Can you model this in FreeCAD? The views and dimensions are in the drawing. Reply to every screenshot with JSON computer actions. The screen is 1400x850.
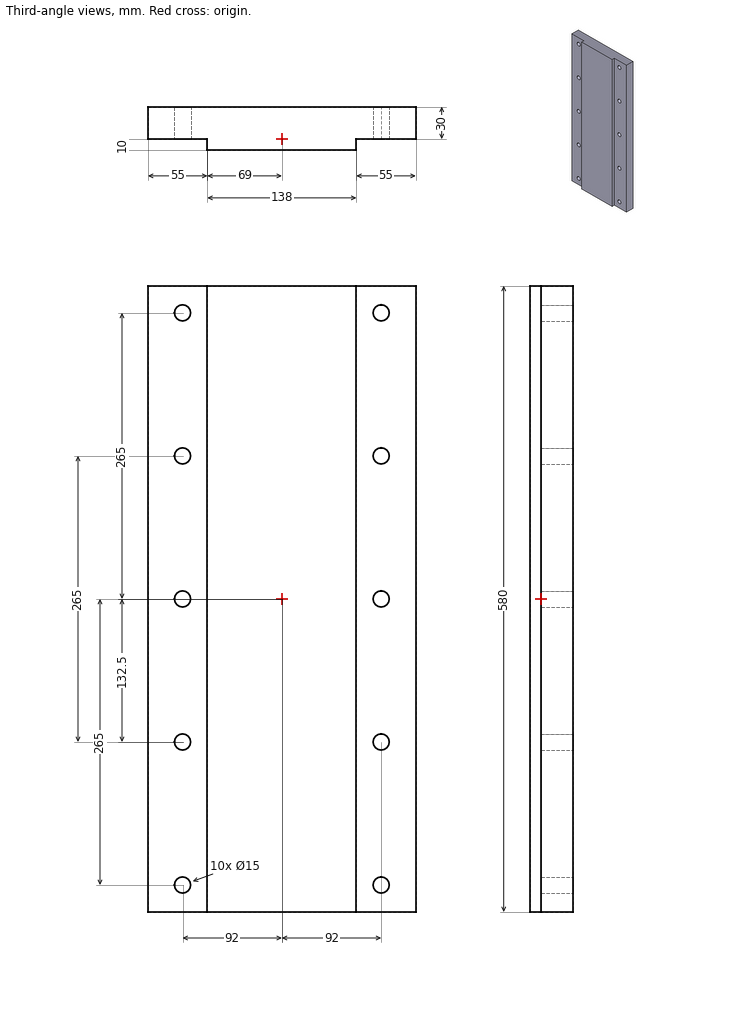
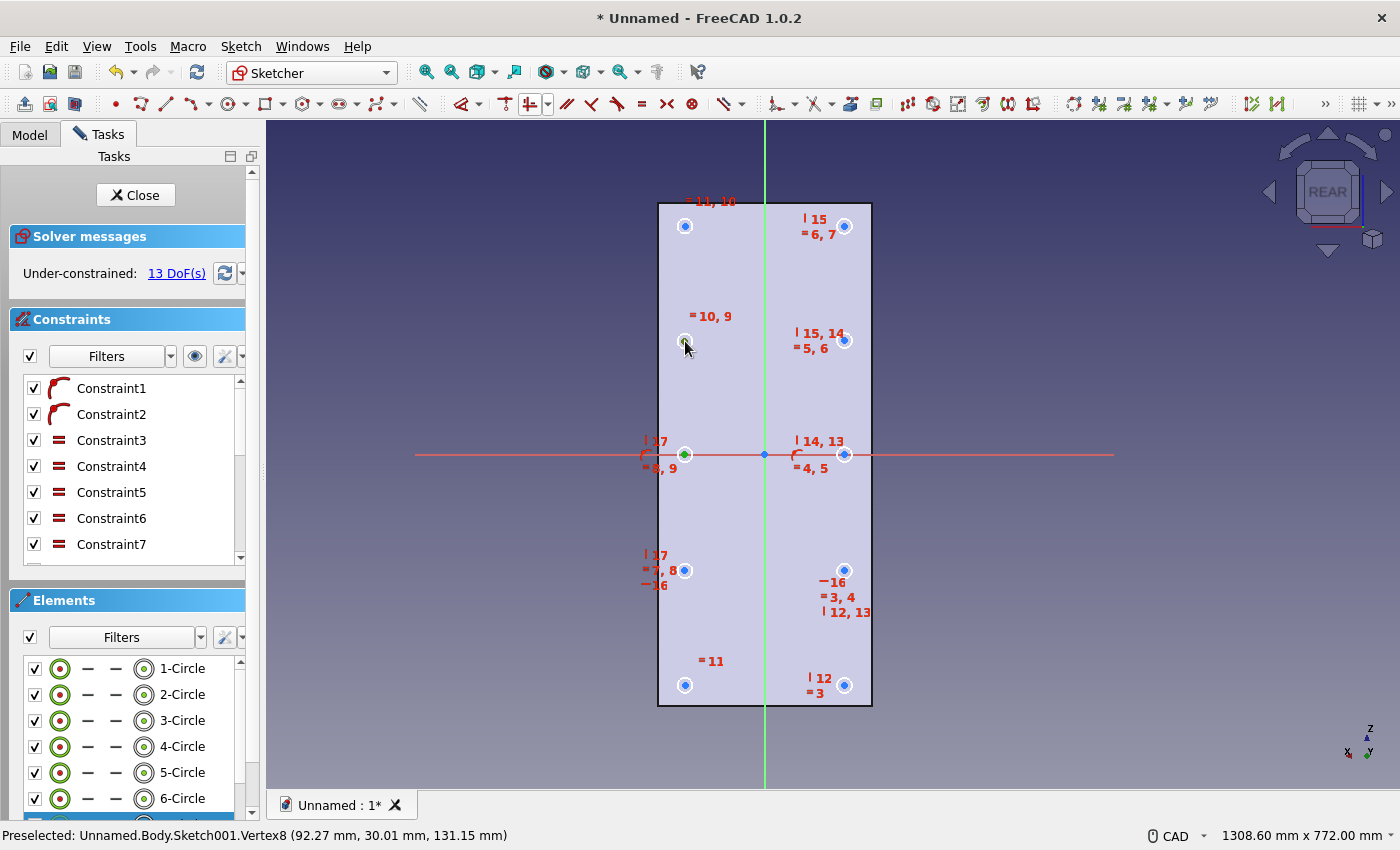
{"action": "left_click", "coordinate": [548, 104]}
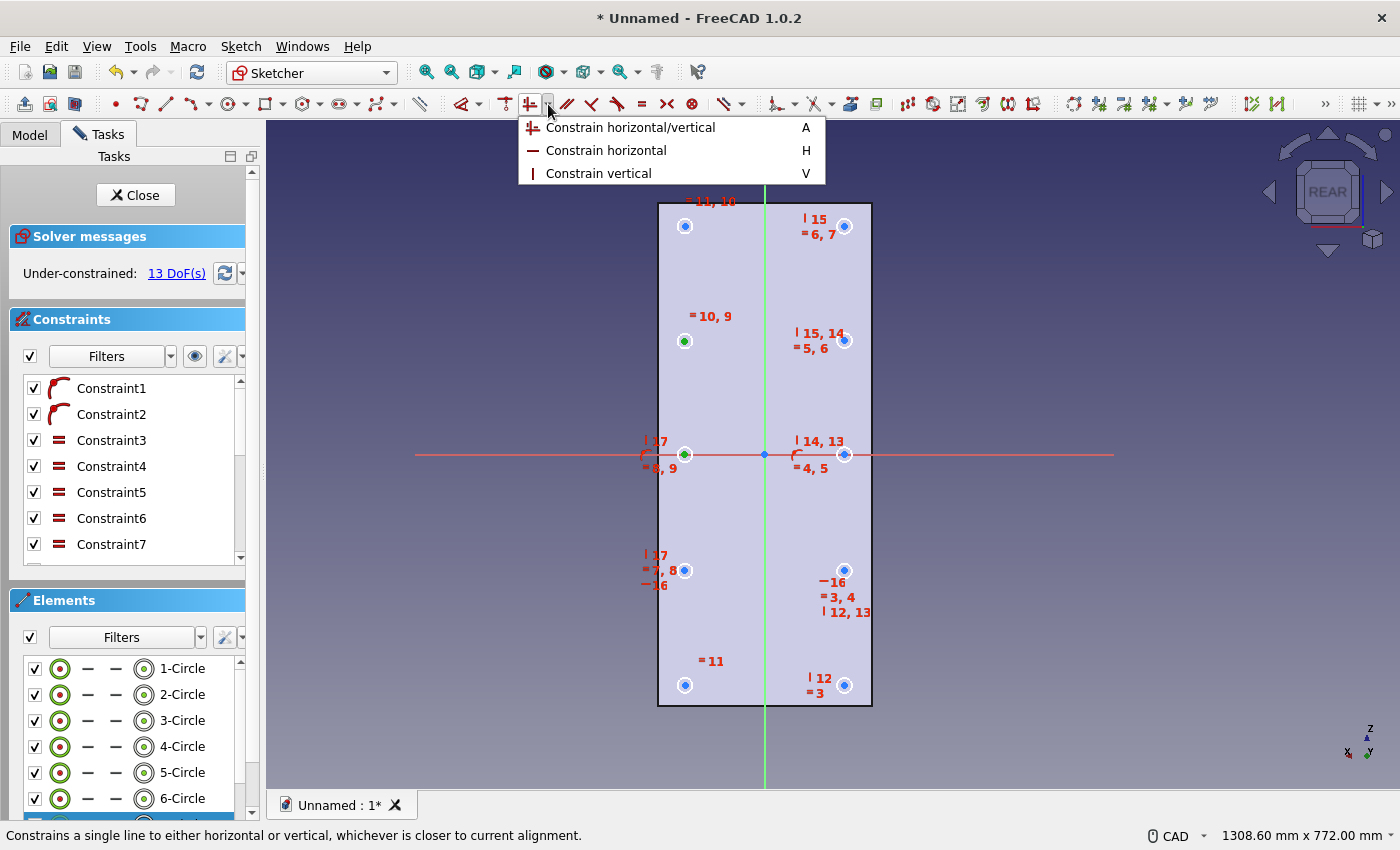
{"action": "left_click", "coordinate": [672, 174]}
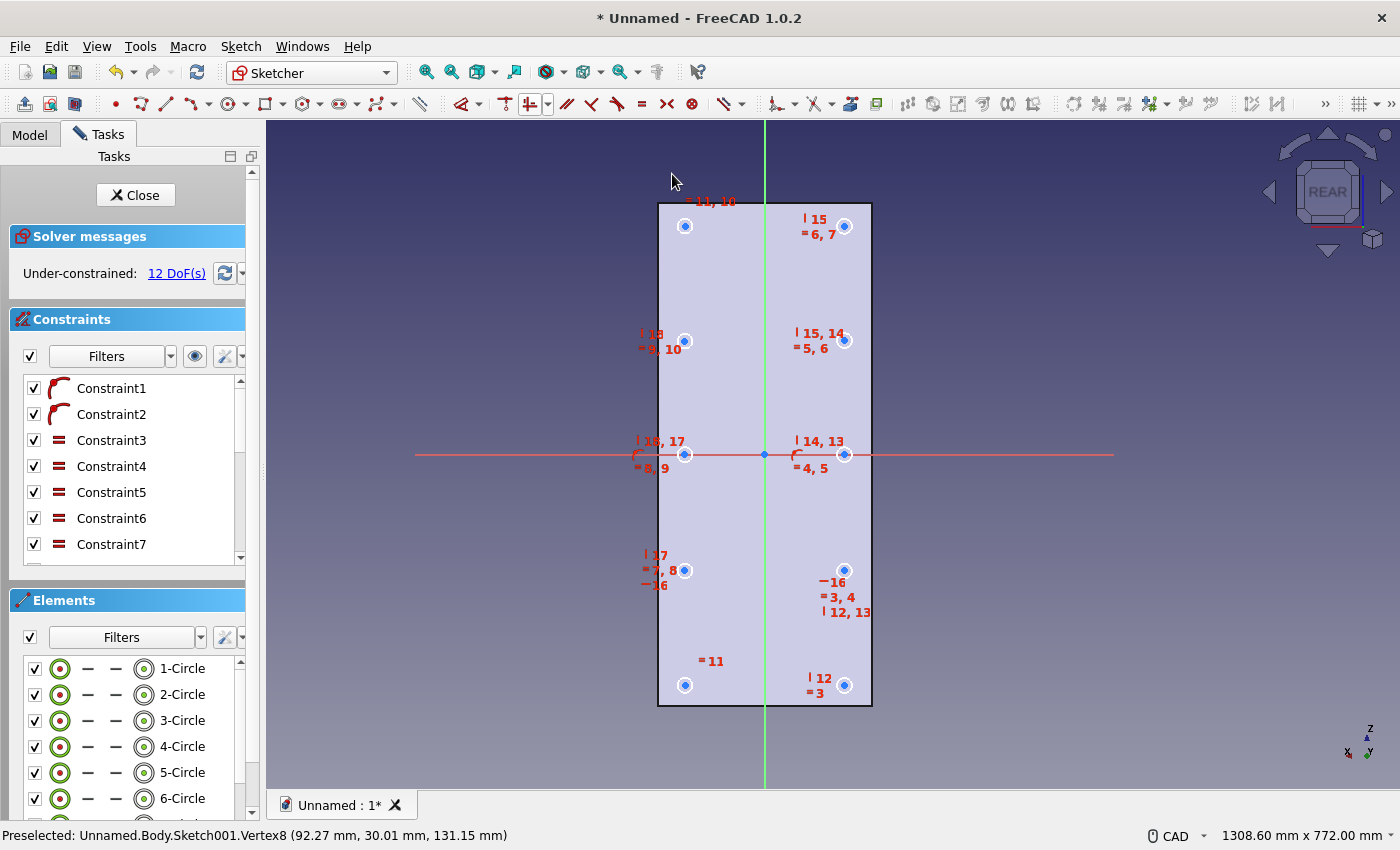
{"action": "left_click", "coordinate": [844, 341]}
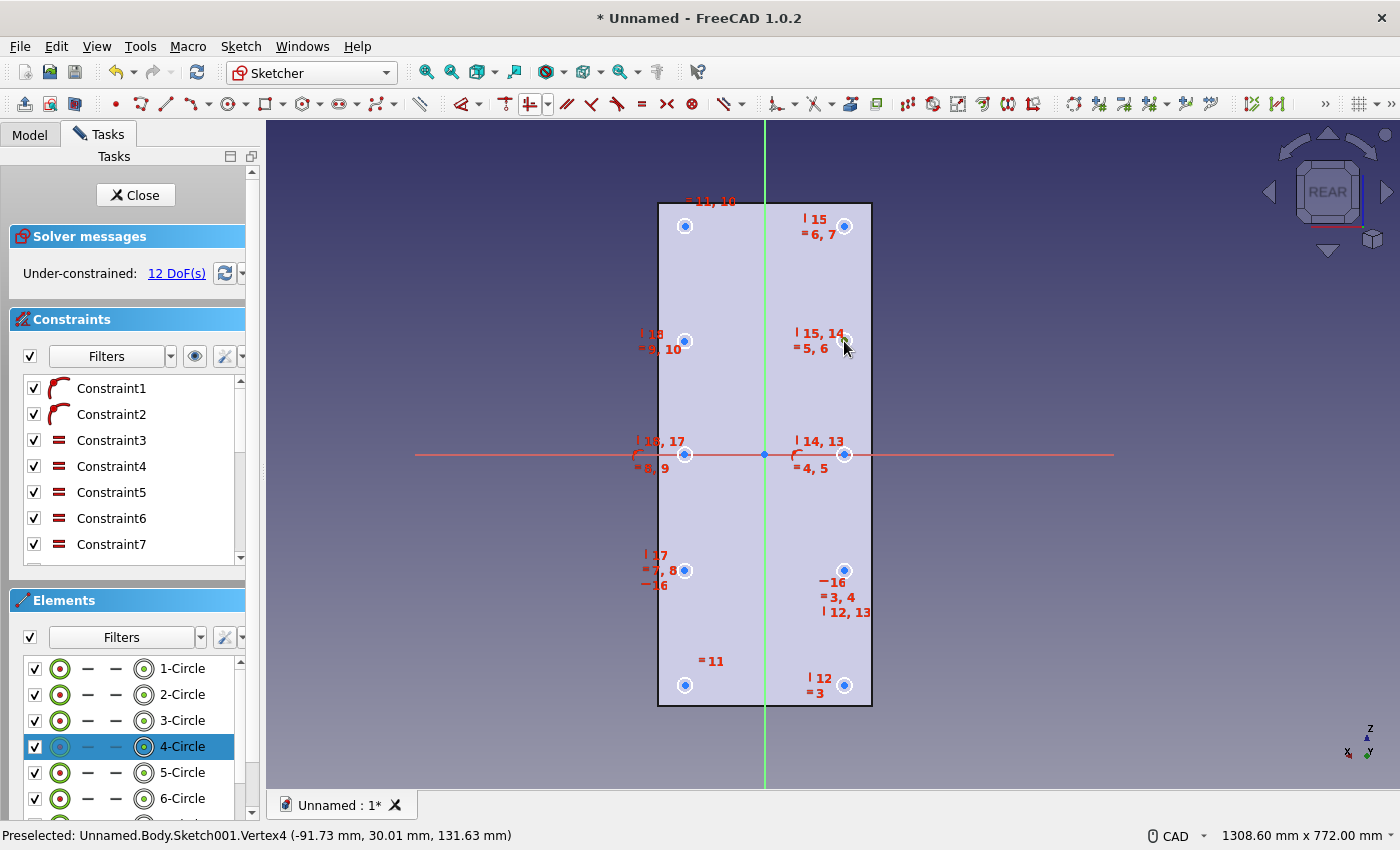
{"action": "left_click", "coordinate": [685, 341]}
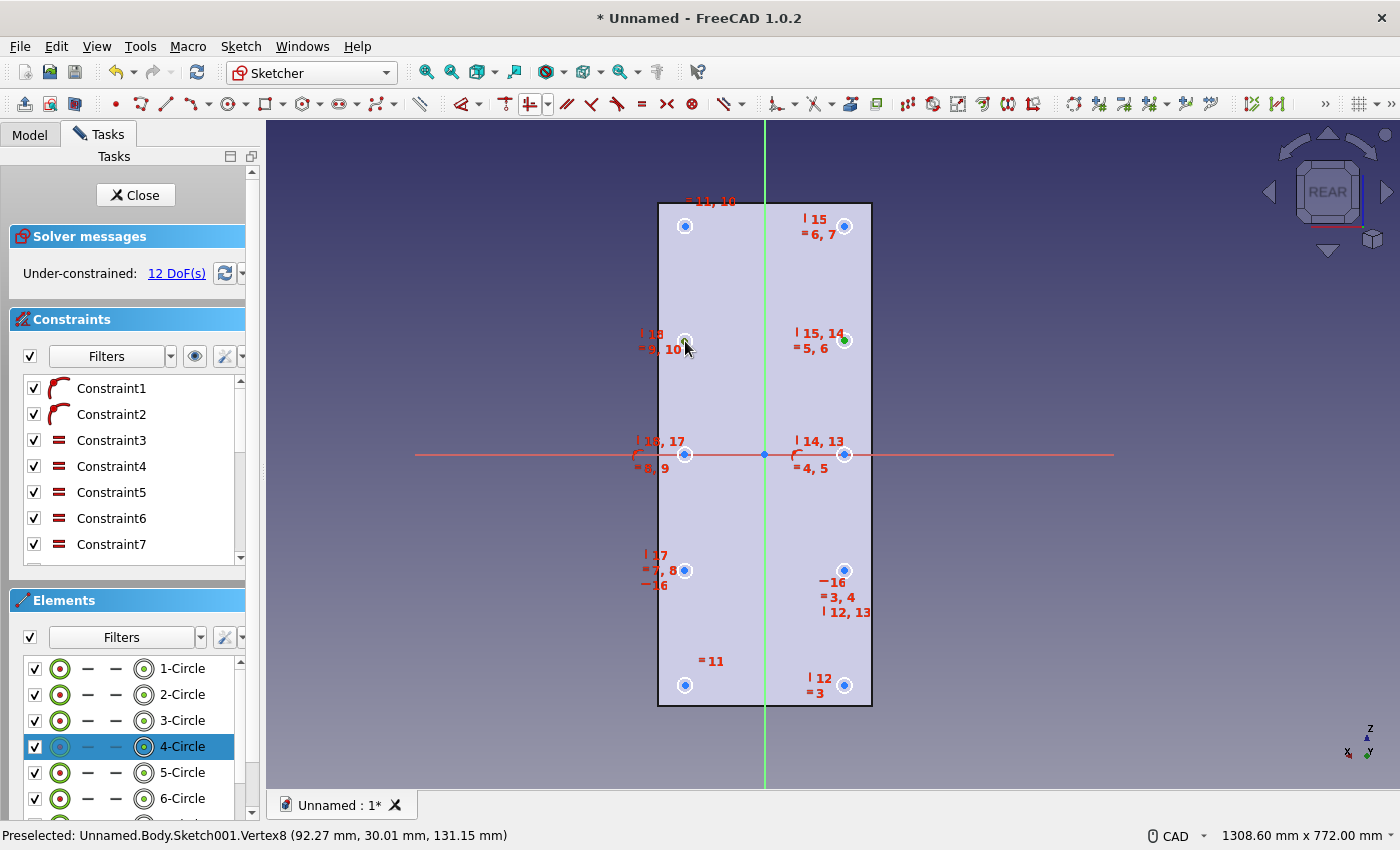
{"action": "key", "text": "h"}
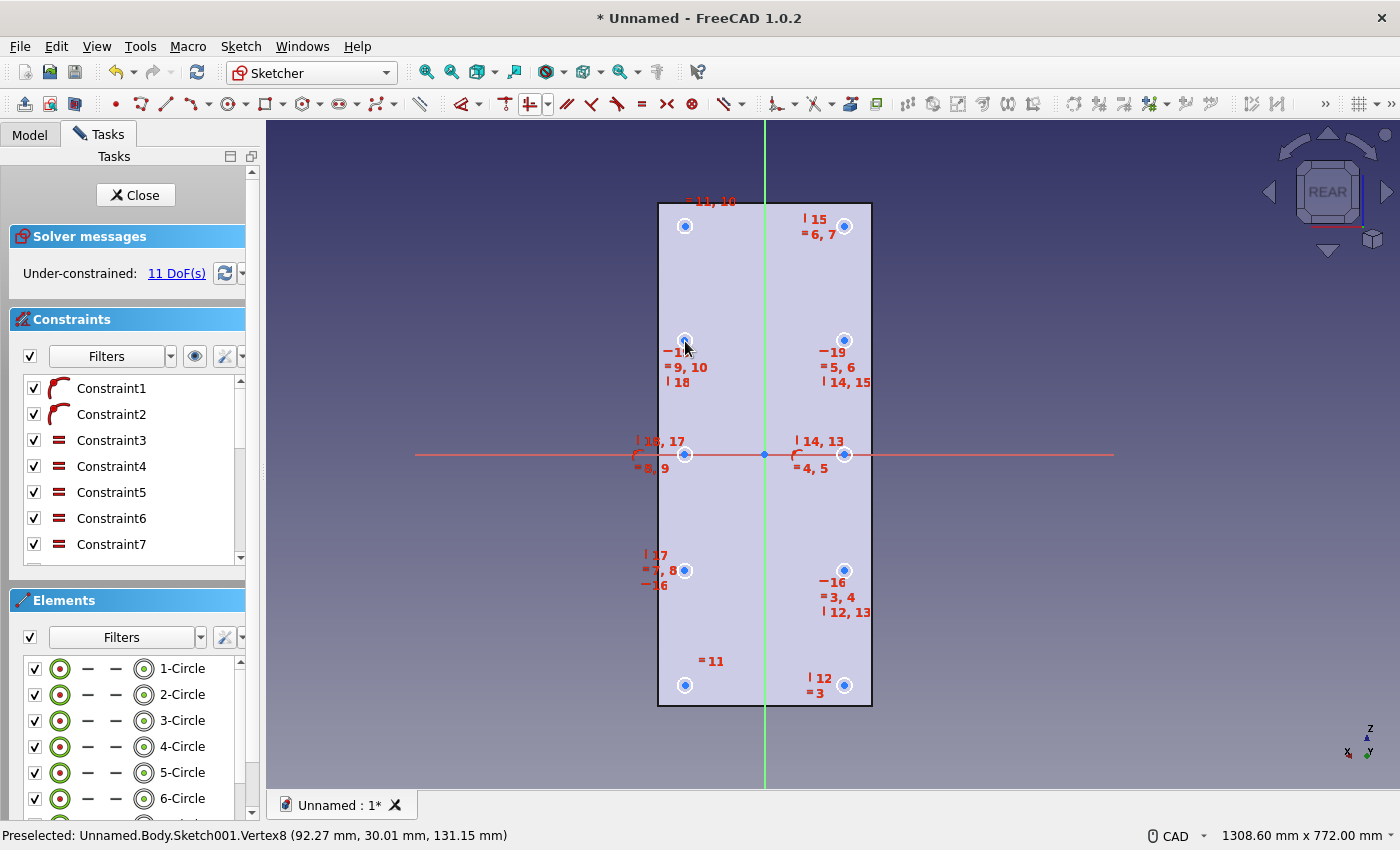
{"action": "left_click", "coordinate": [685, 341]}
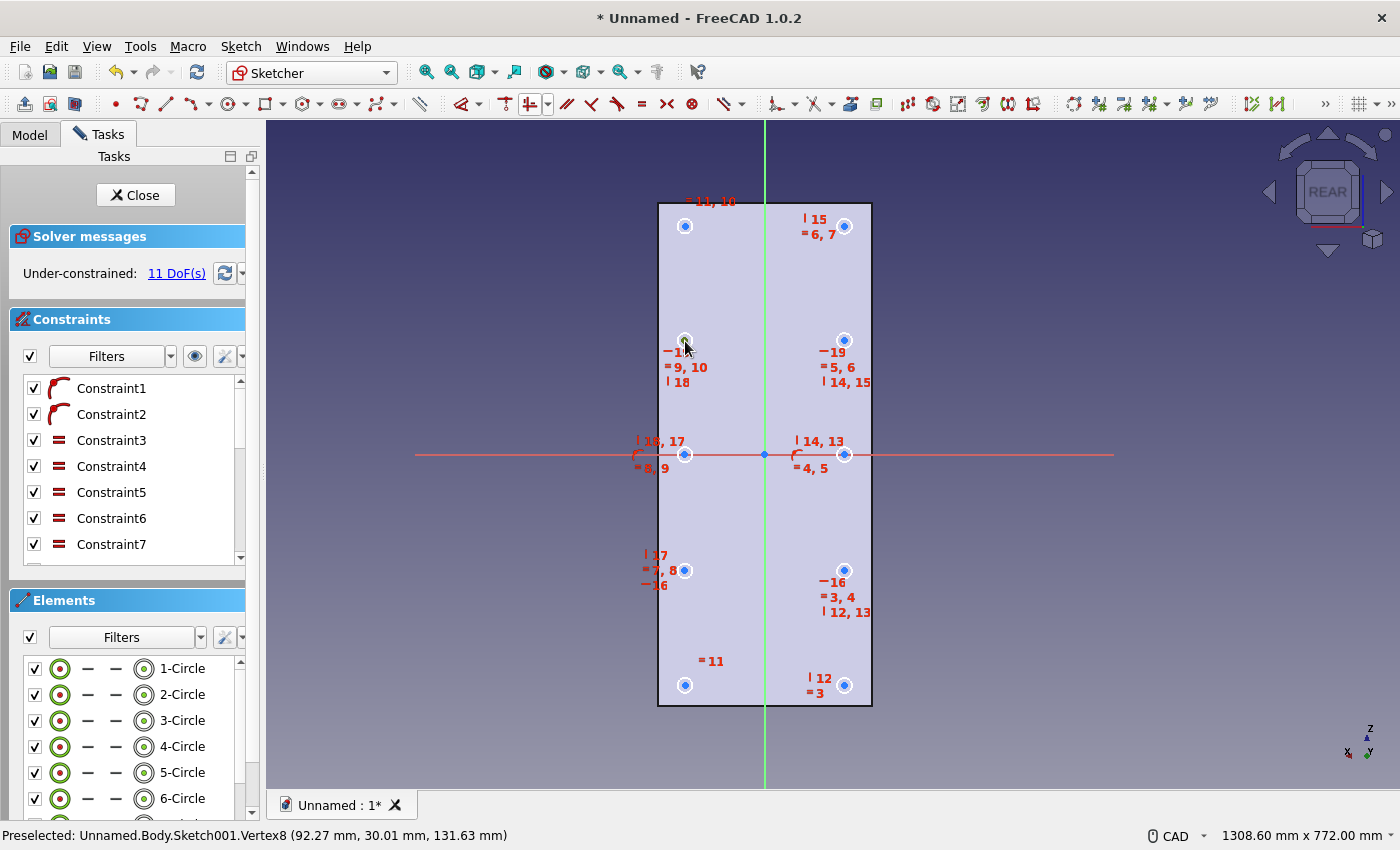
{"action": "left_click", "coordinate": [685, 226]}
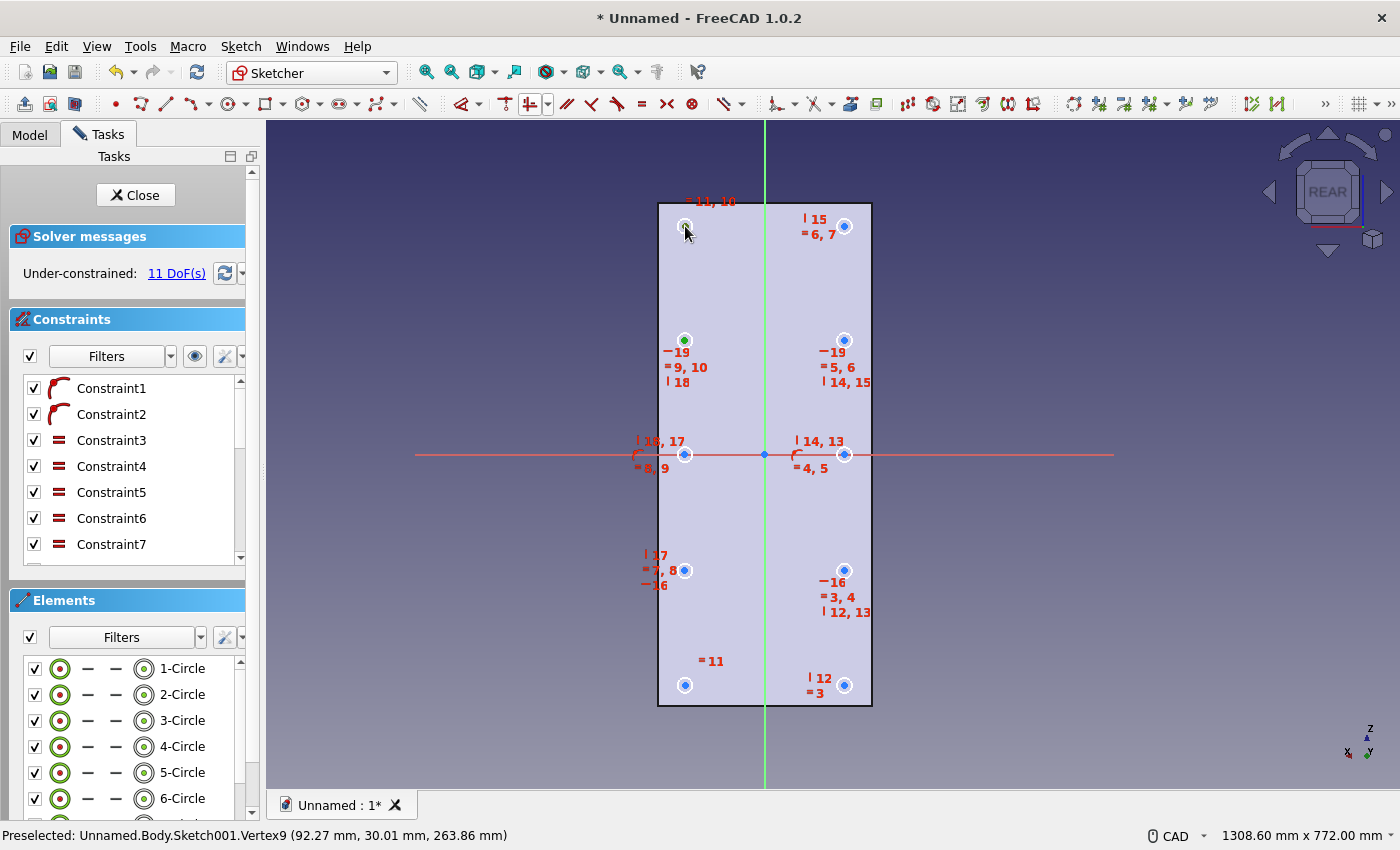
{"action": "left_click", "coordinate": [548, 104]}